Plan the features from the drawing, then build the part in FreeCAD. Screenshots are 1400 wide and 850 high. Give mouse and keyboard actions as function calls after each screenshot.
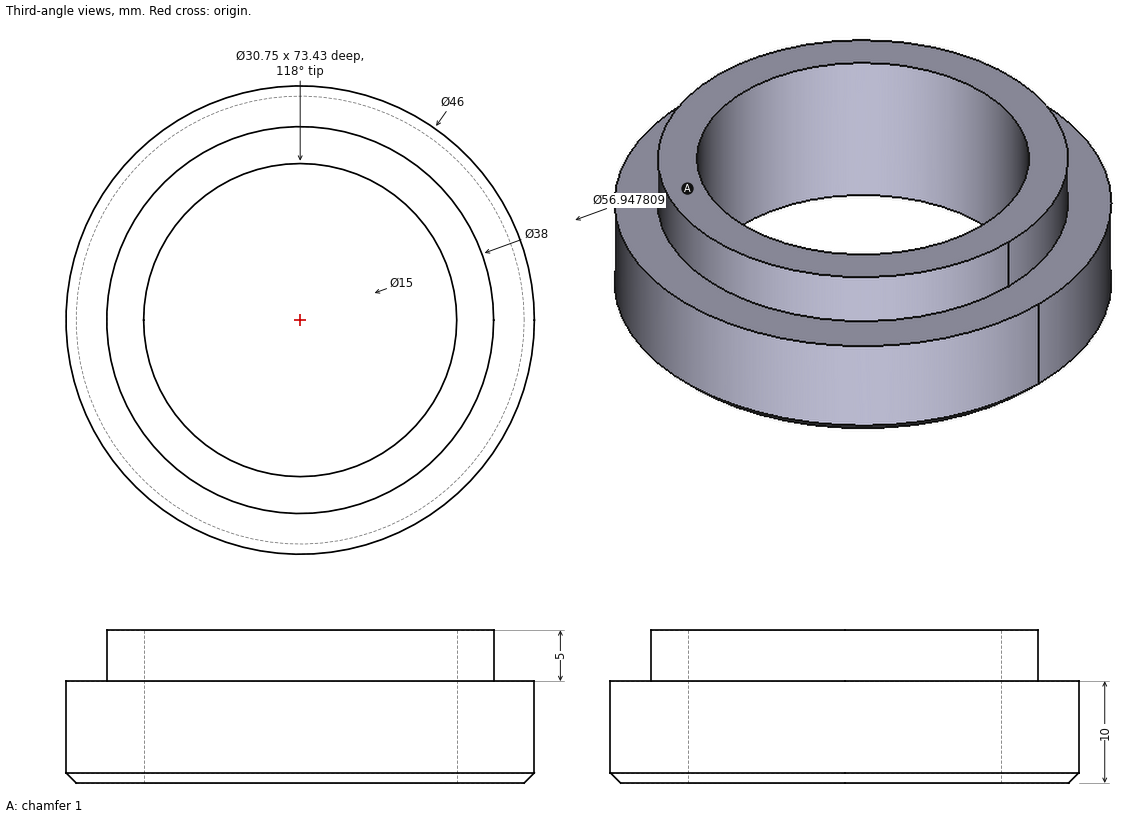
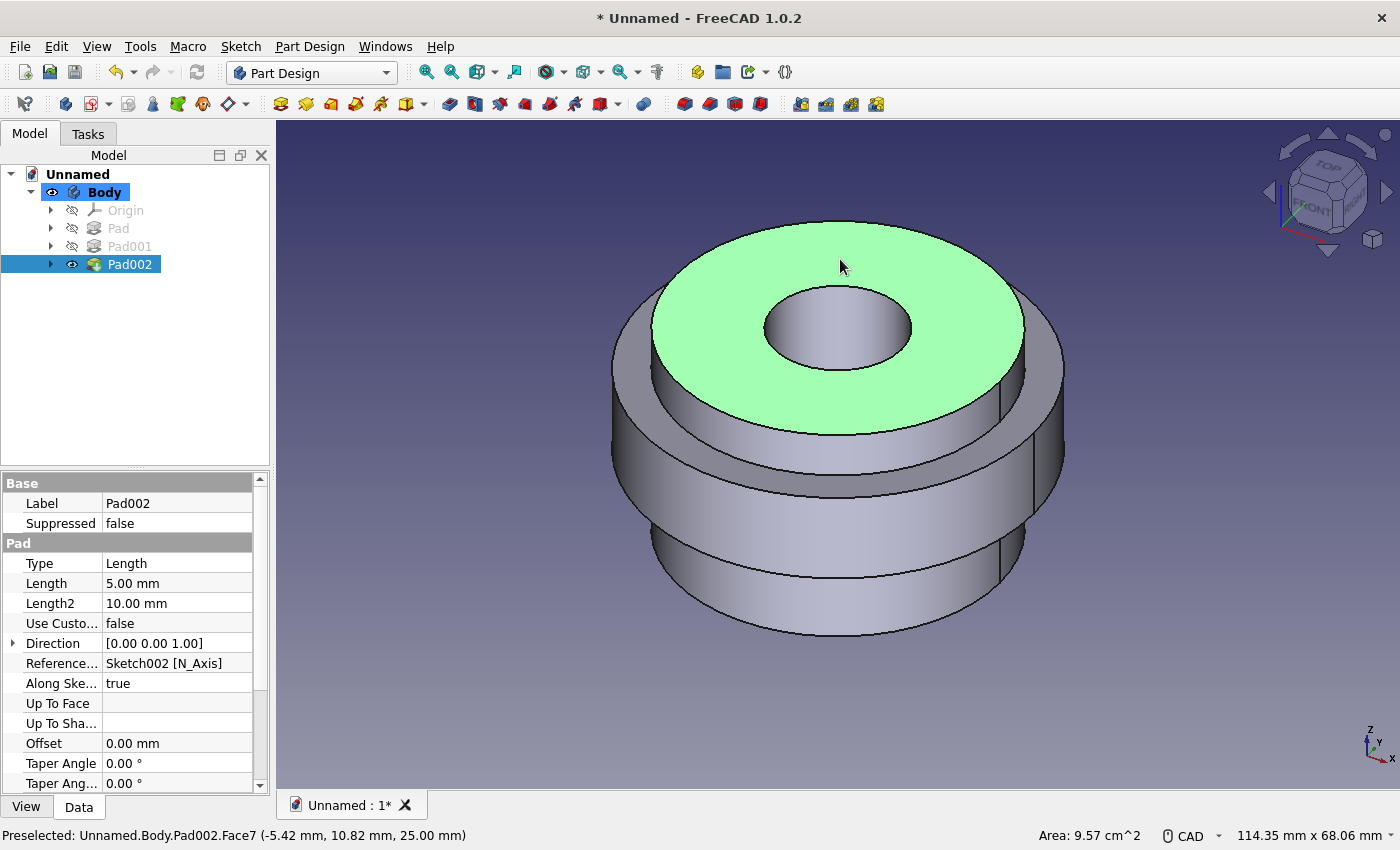
click(90, 104)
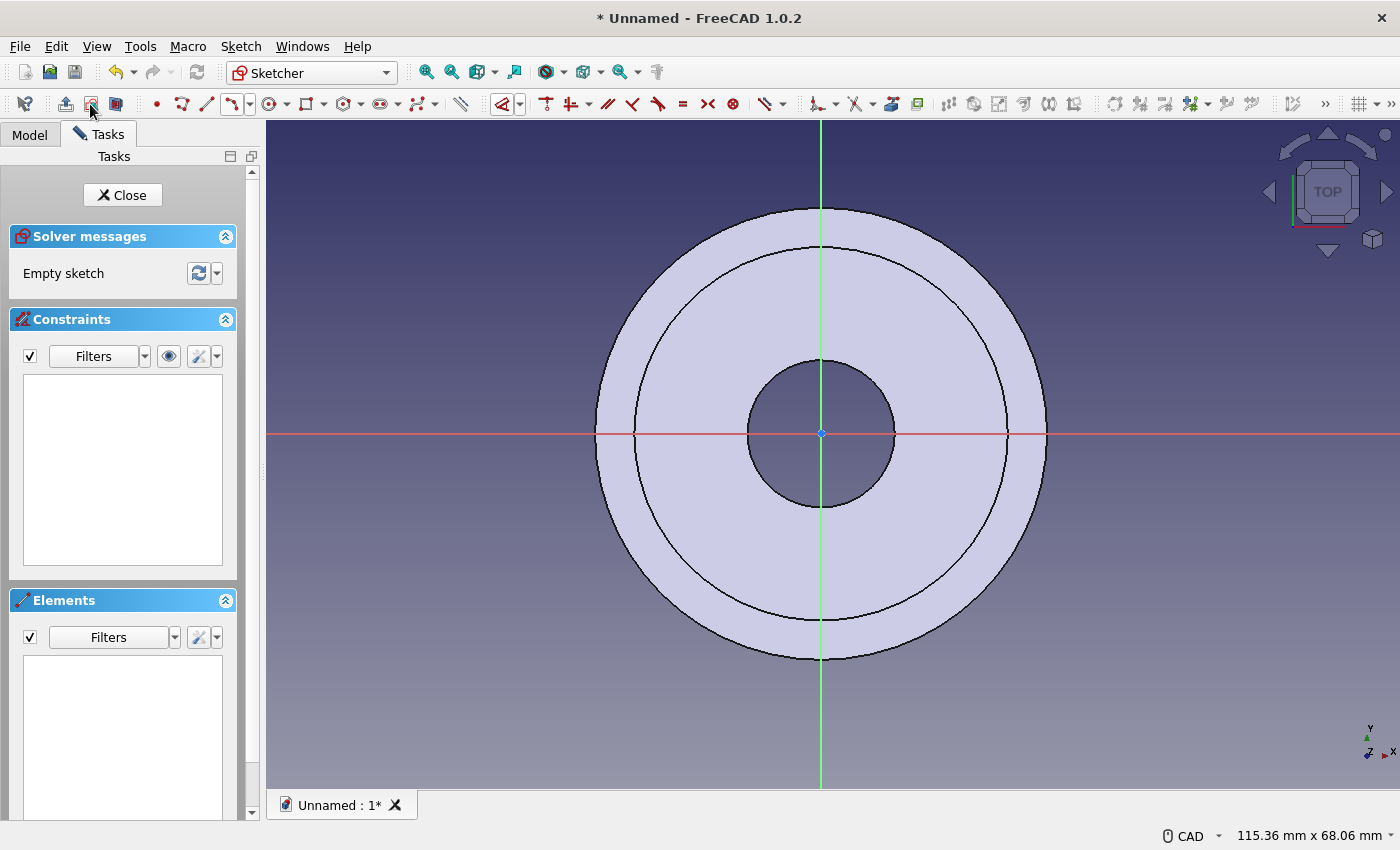
scroll(936, 392, up, 2)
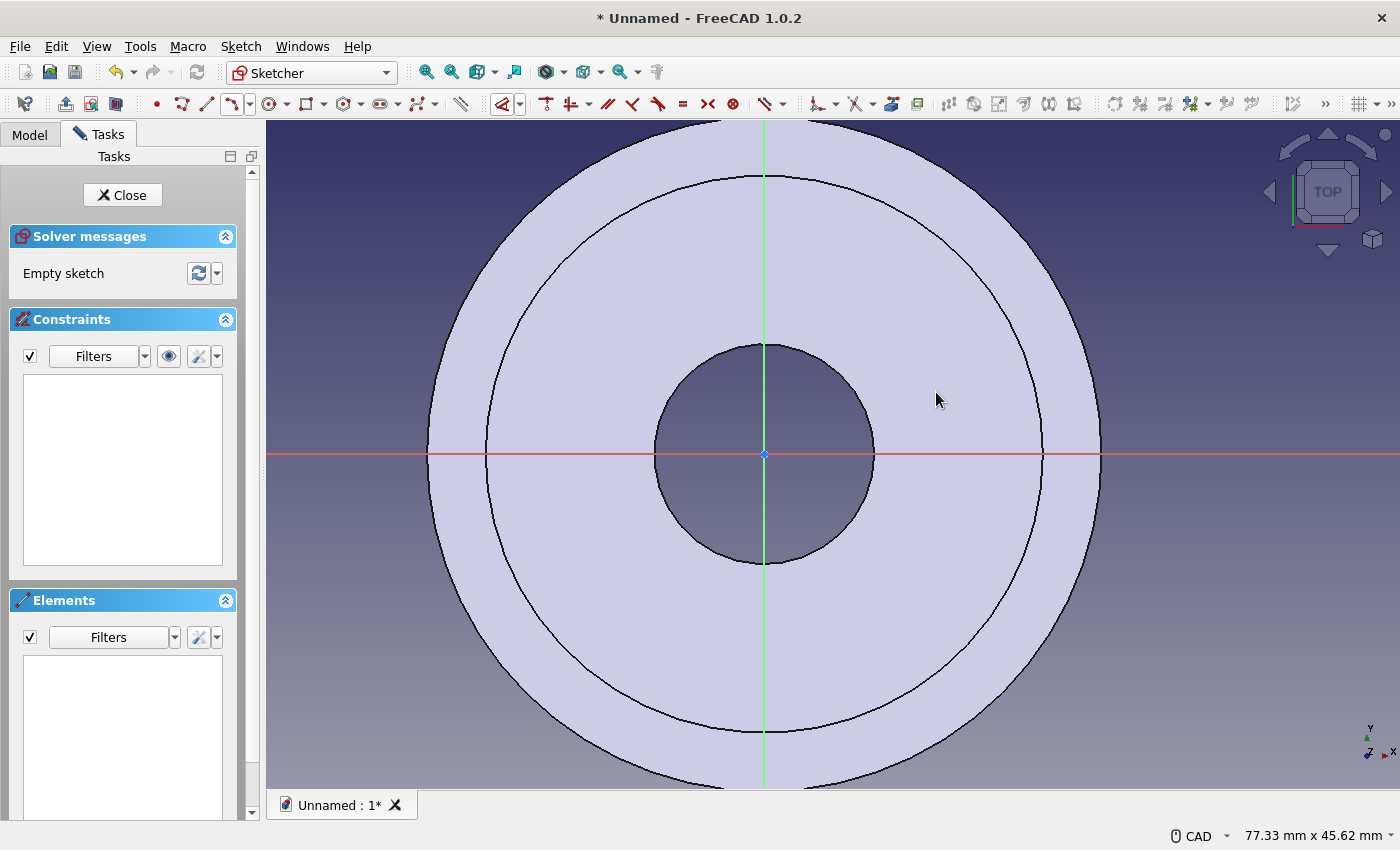
click(268, 104)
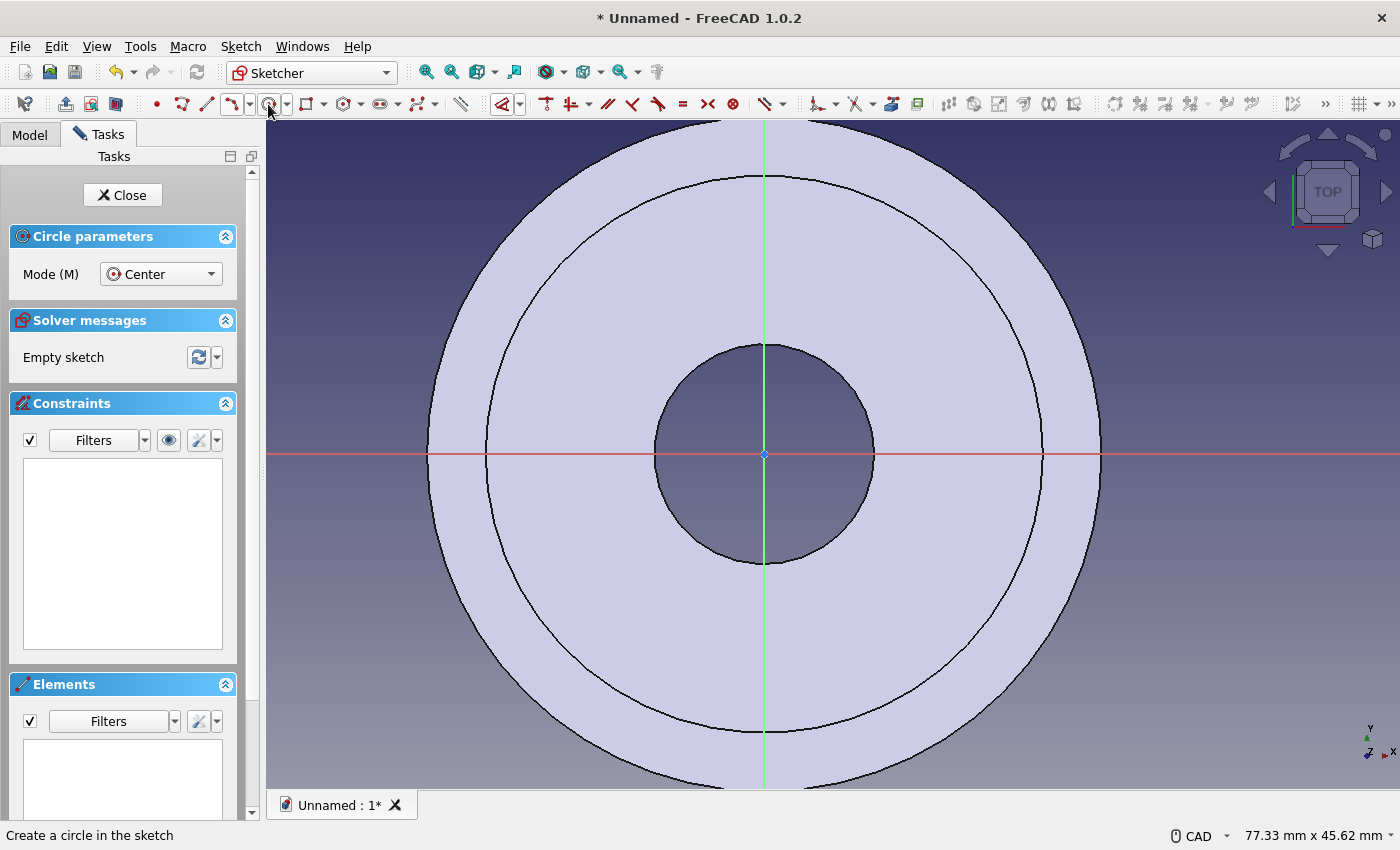
click(764, 454)
move(924, 295)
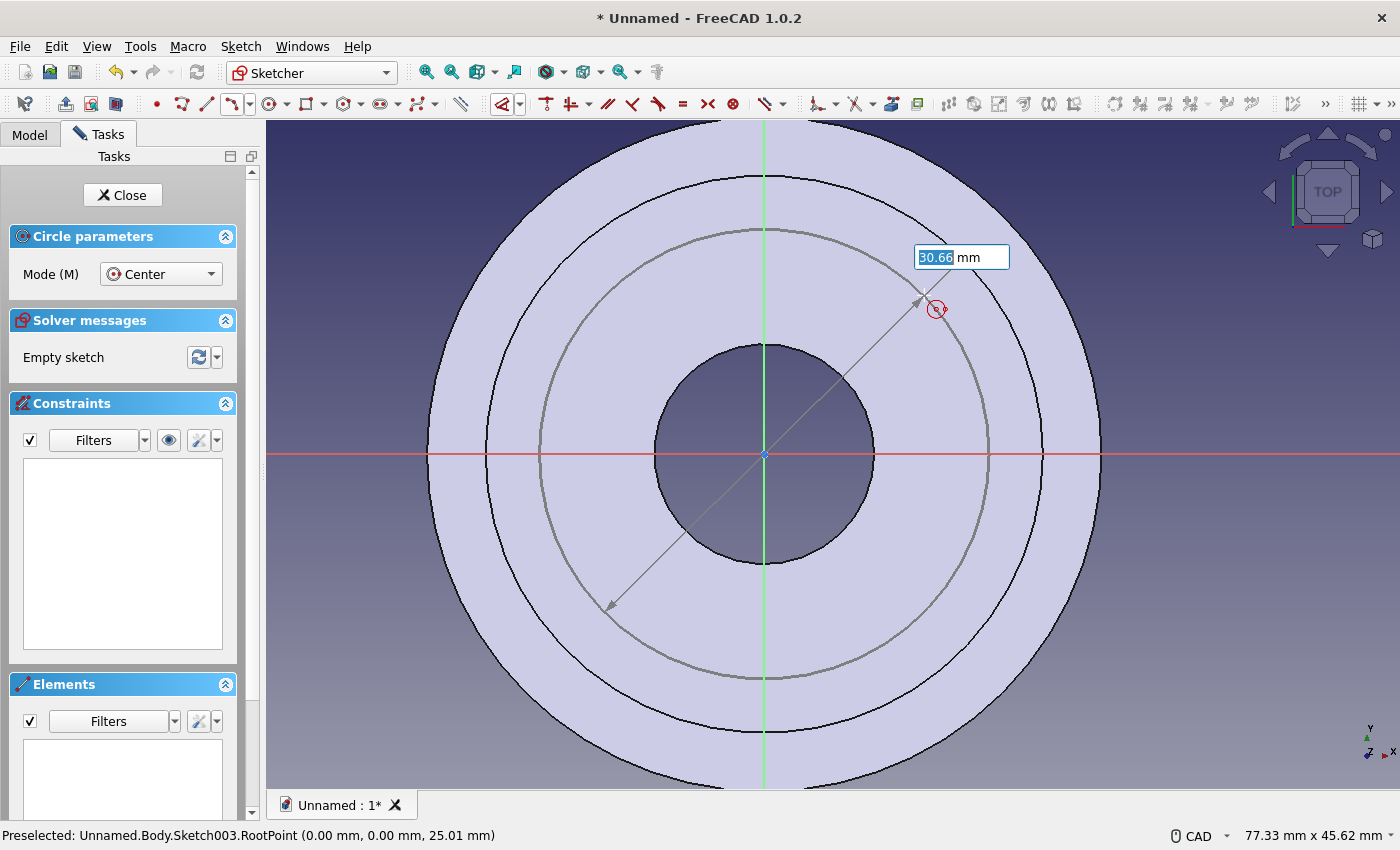
text(30.75)
key(Return)
key(Escape)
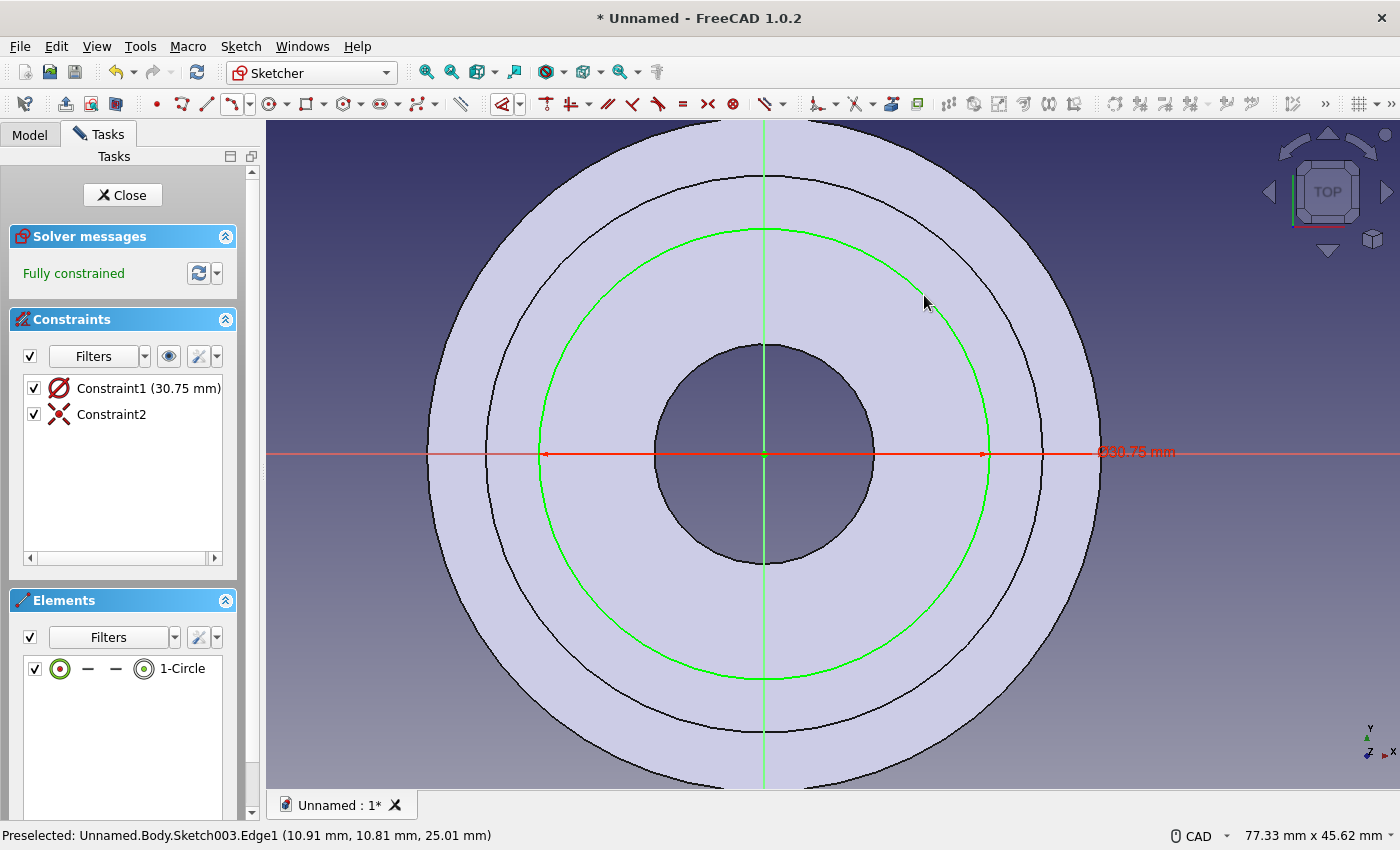
click(123, 195)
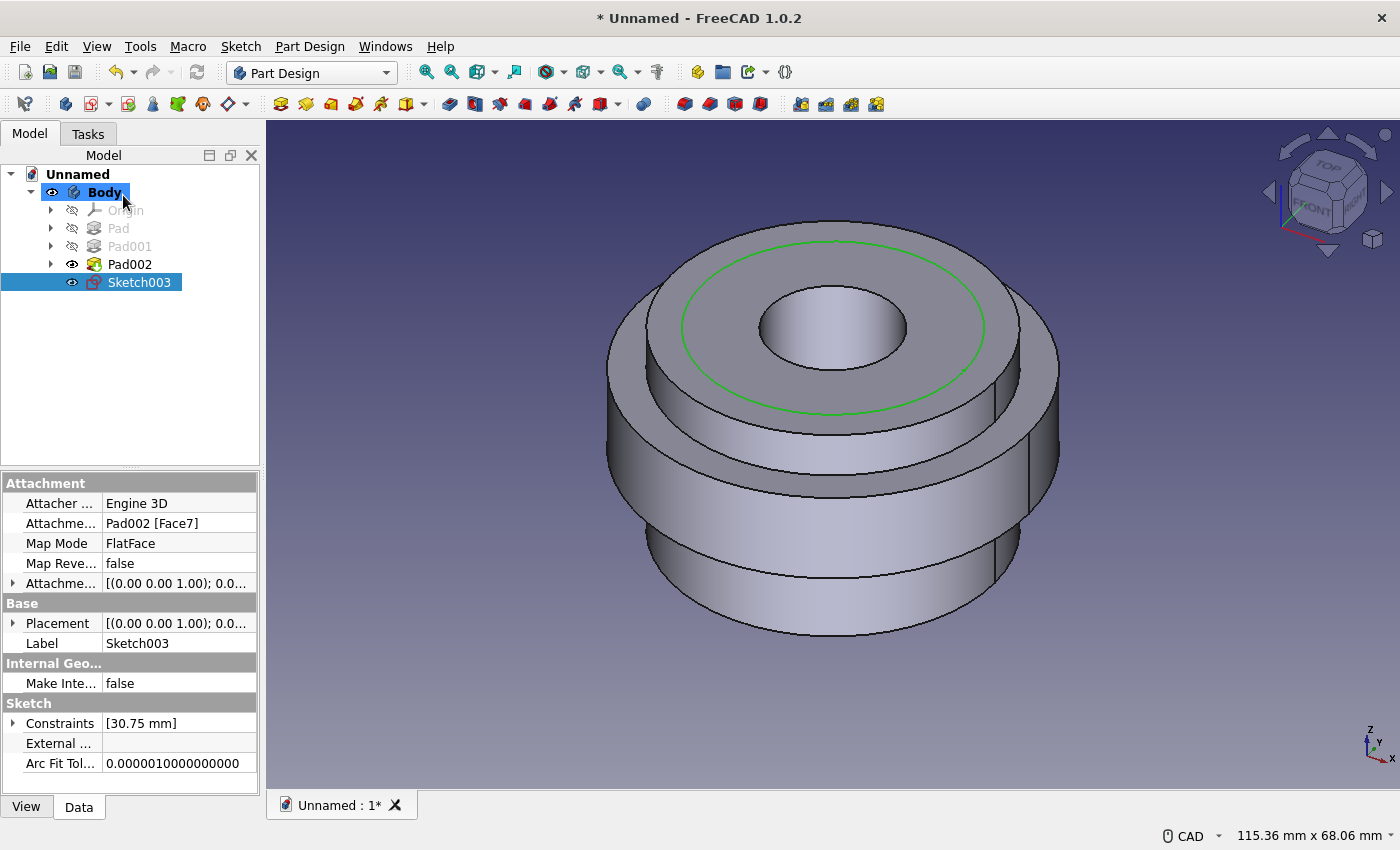
click(475, 104)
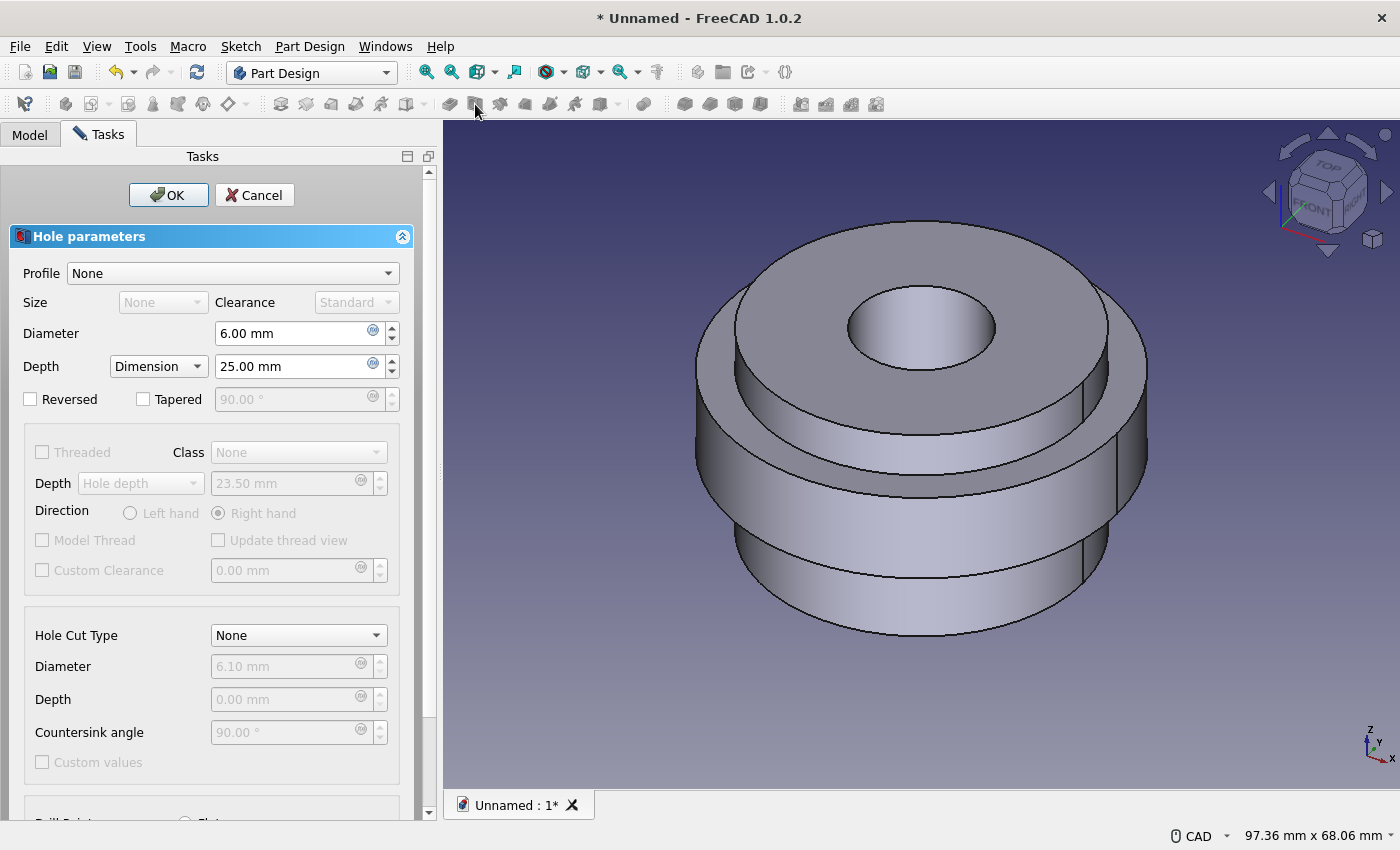
triple_click(300, 334)